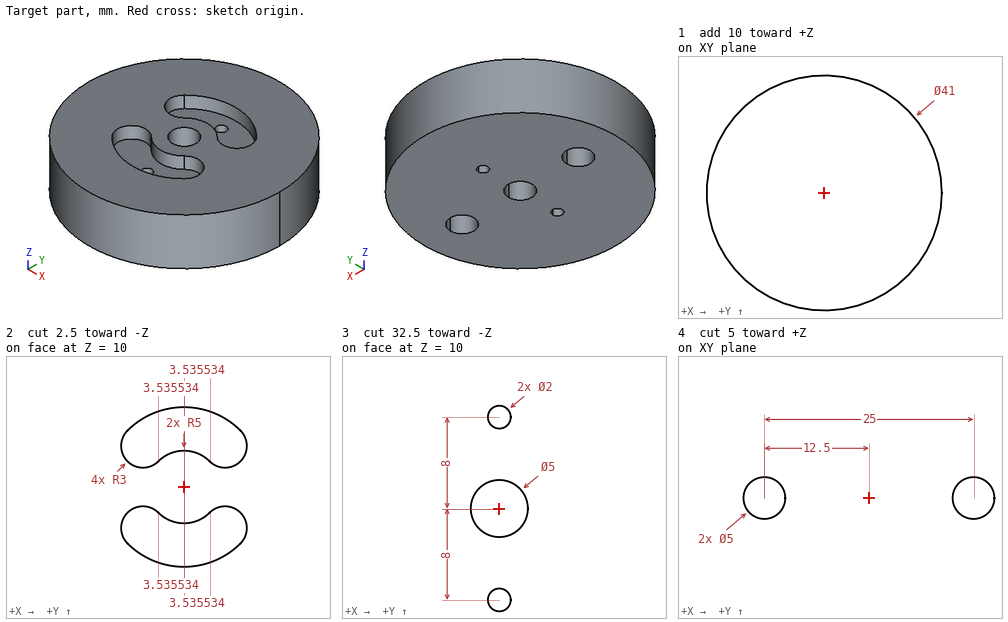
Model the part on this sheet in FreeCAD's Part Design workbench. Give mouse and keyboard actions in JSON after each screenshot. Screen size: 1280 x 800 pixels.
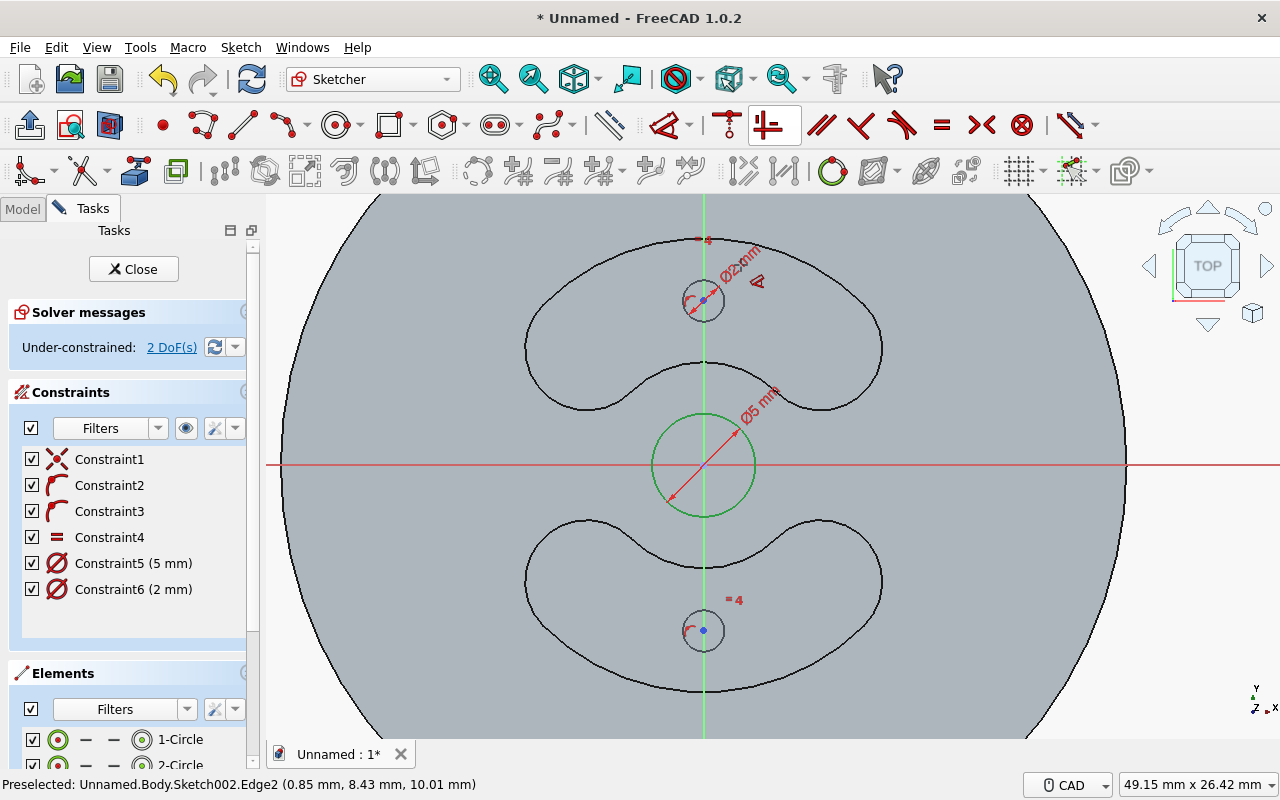
{"action": "left_click", "coordinate": [704, 301]}
{"action": "left_click", "coordinate": [738, 383]}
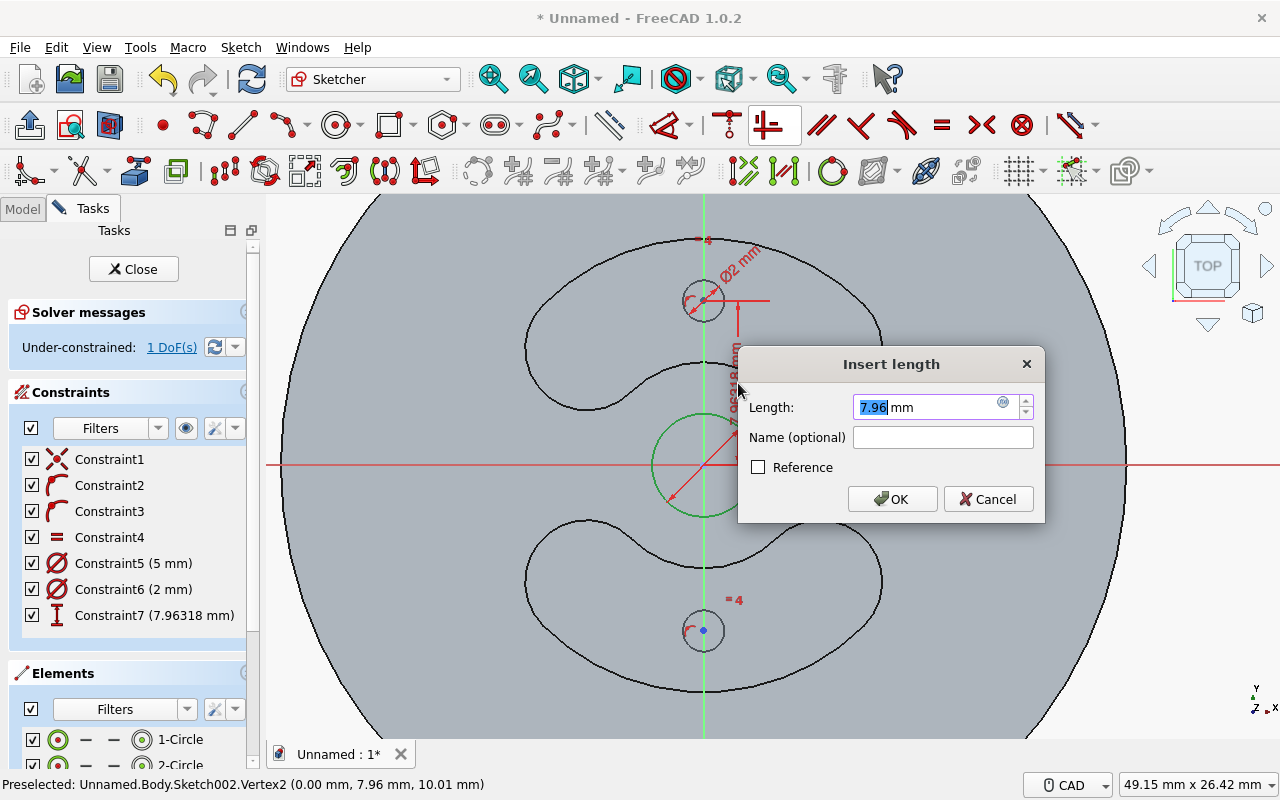
{"action": "type", "text": "8"}
{"action": "key", "text": "Return"}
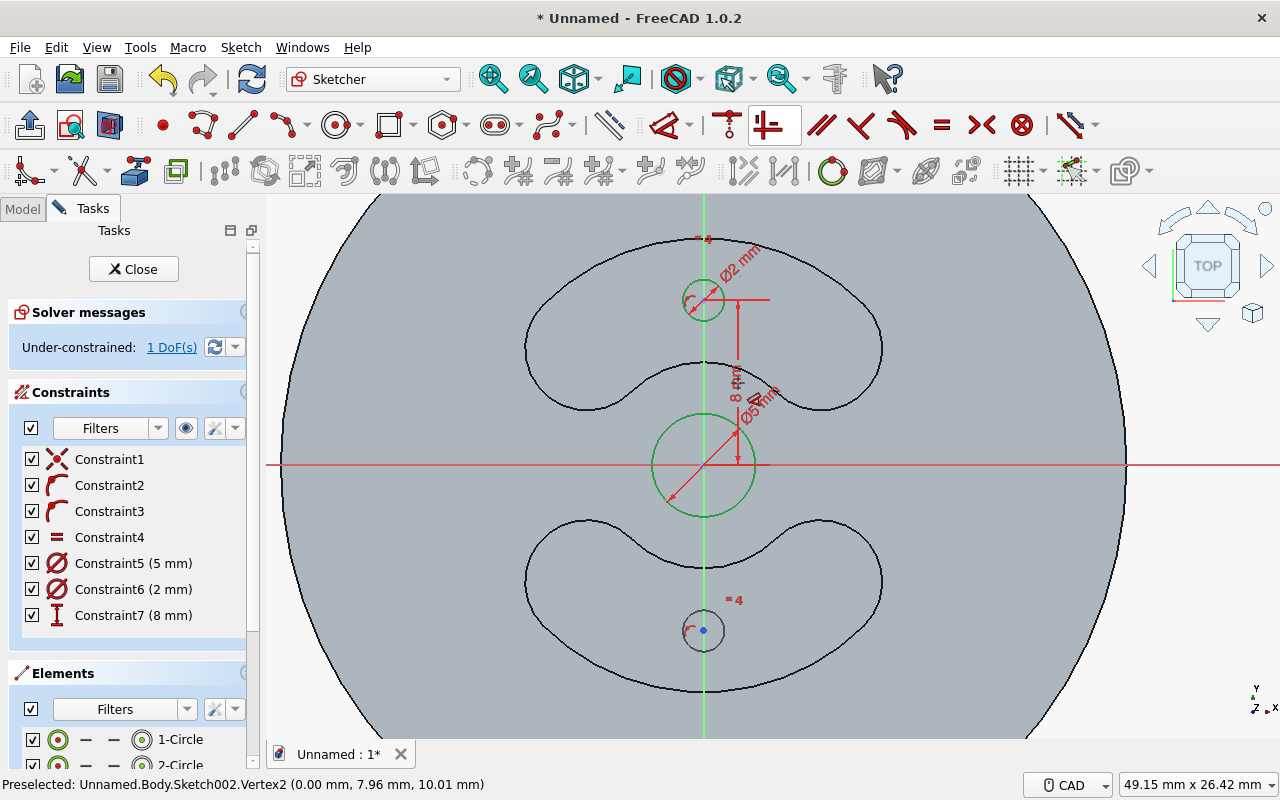
{"action": "left_click", "coordinate": [704, 631]}
{"action": "left_click", "coordinate": [738, 548]}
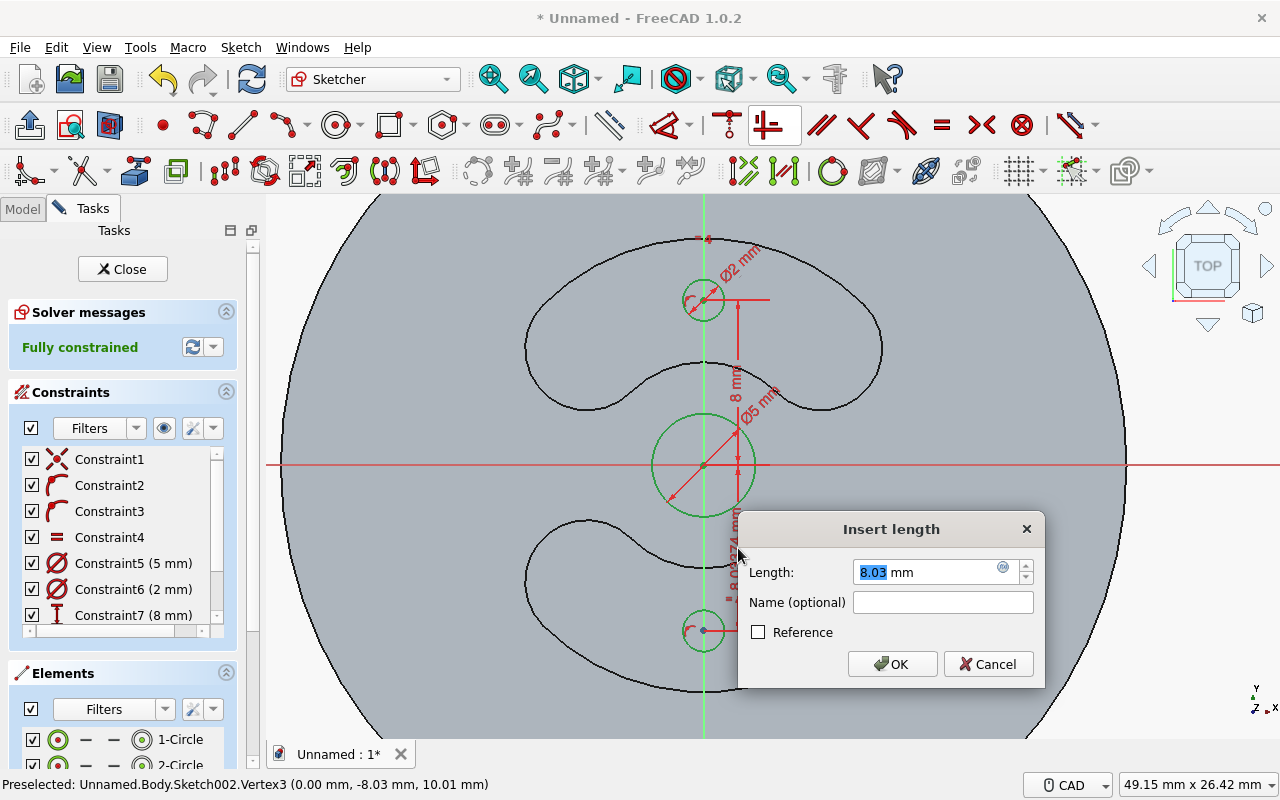
{"action": "type", "text": "8"}
{"action": "key", "text": "Return"}
{"action": "key", "text": "Escape"}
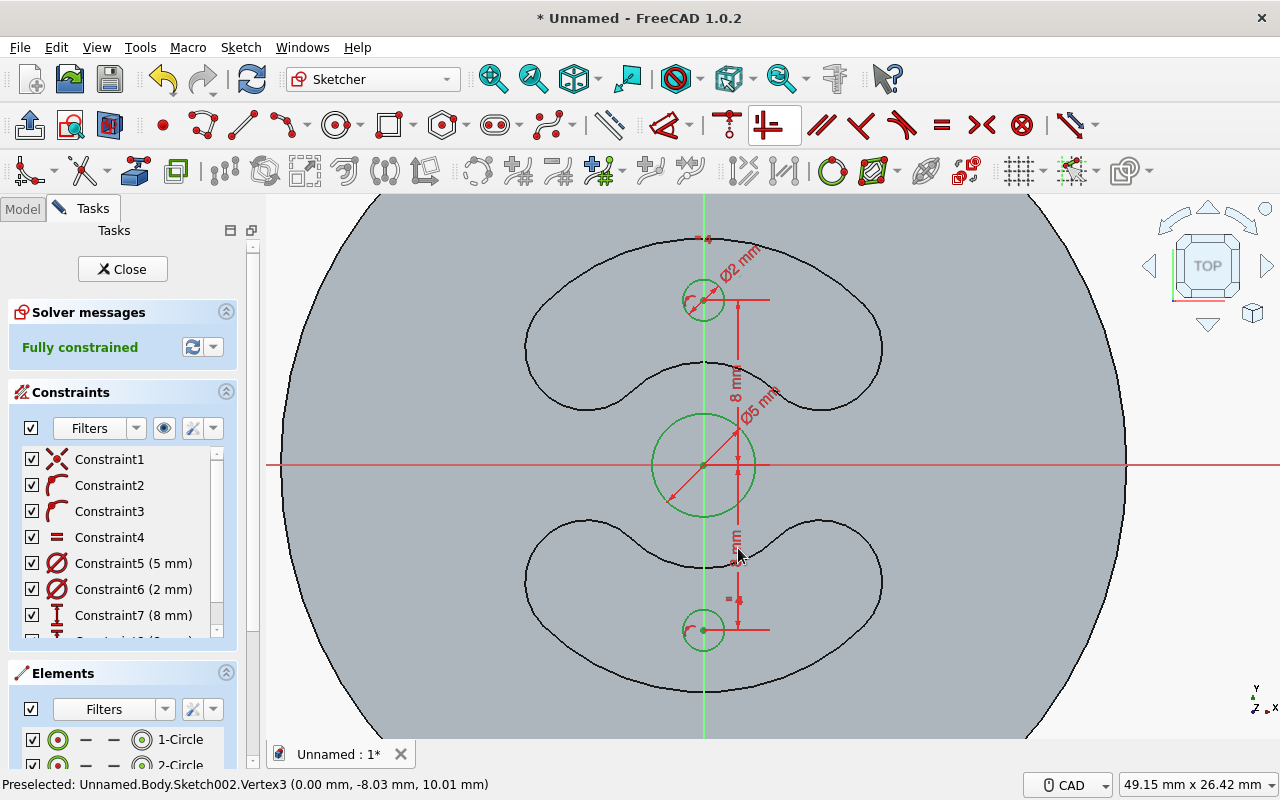
{"action": "left_click", "coordinate": [123, 269]}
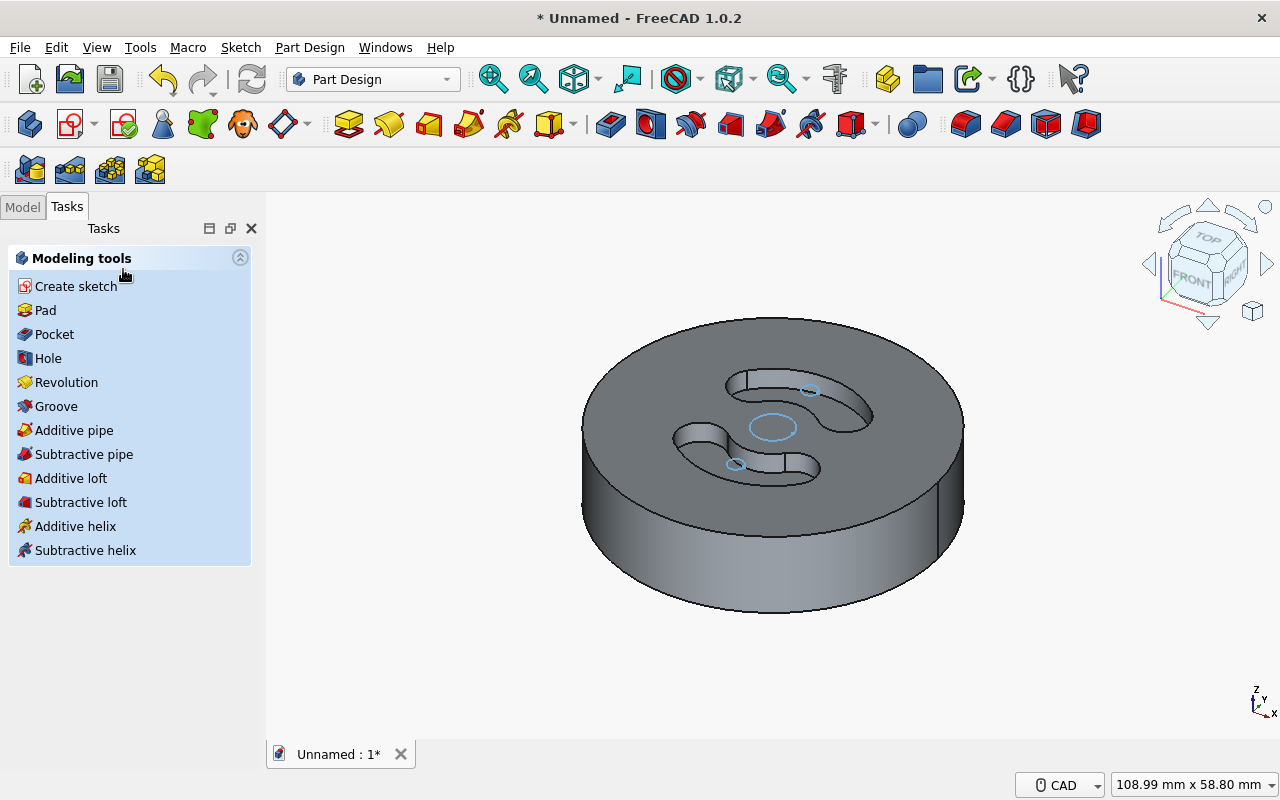
{"action": "left_click", "coordinate": [612, 124]}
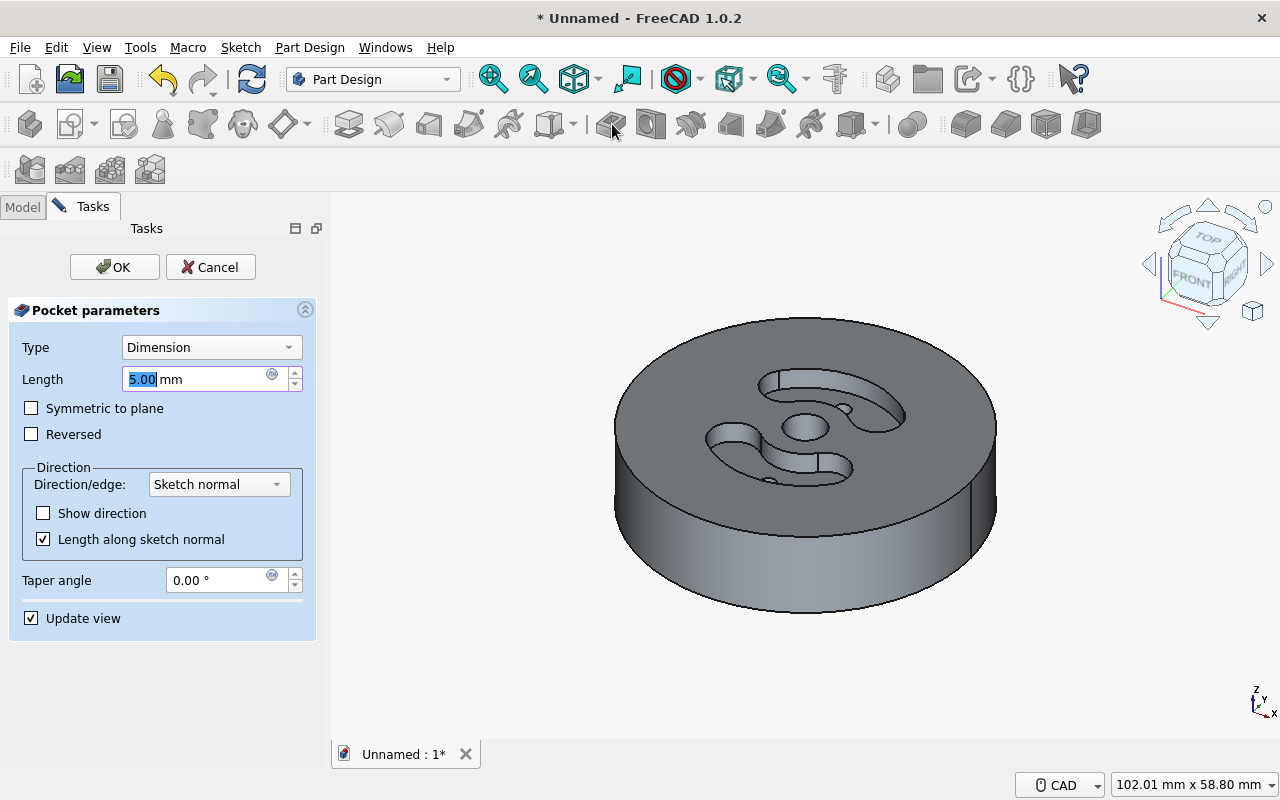
{"action": "type", "text": "32.5"}
{"action": "key", "text": "Tab"}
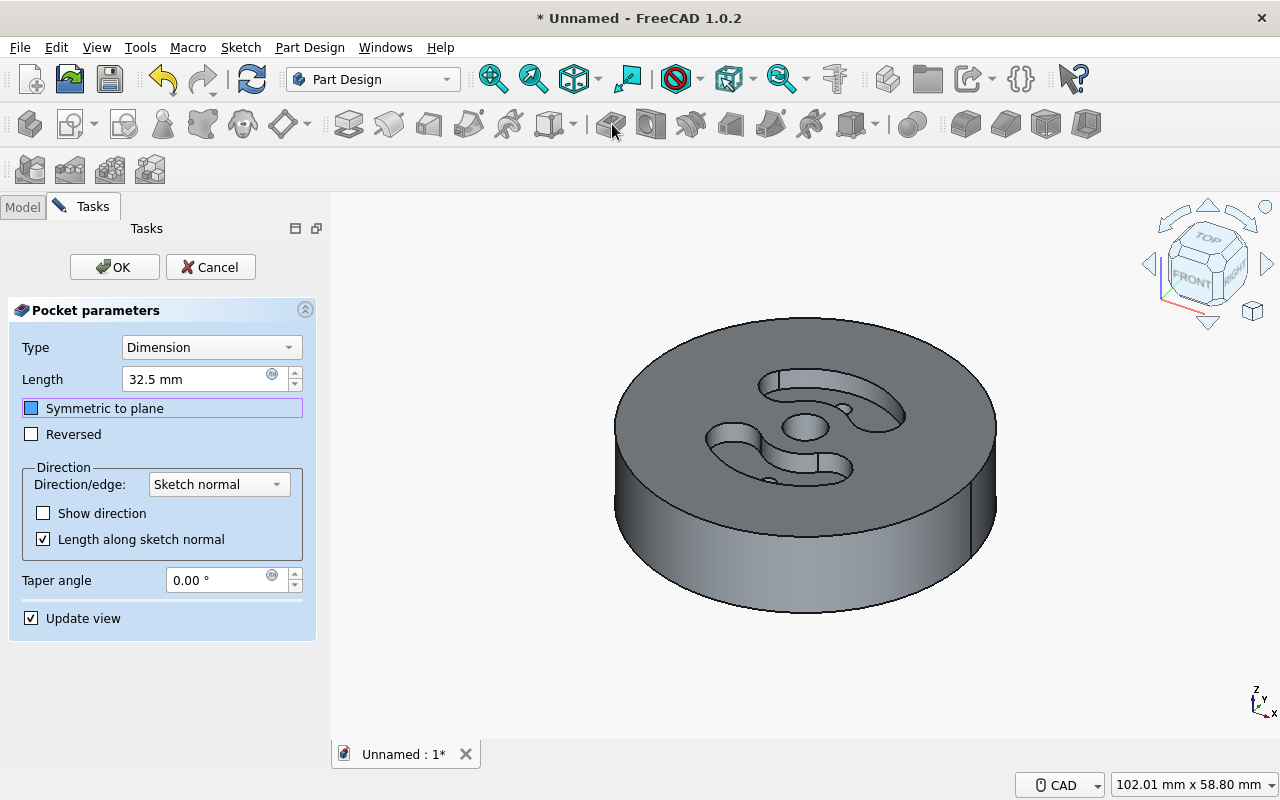
{"action": "left_click", "coordinate": [115, 267]}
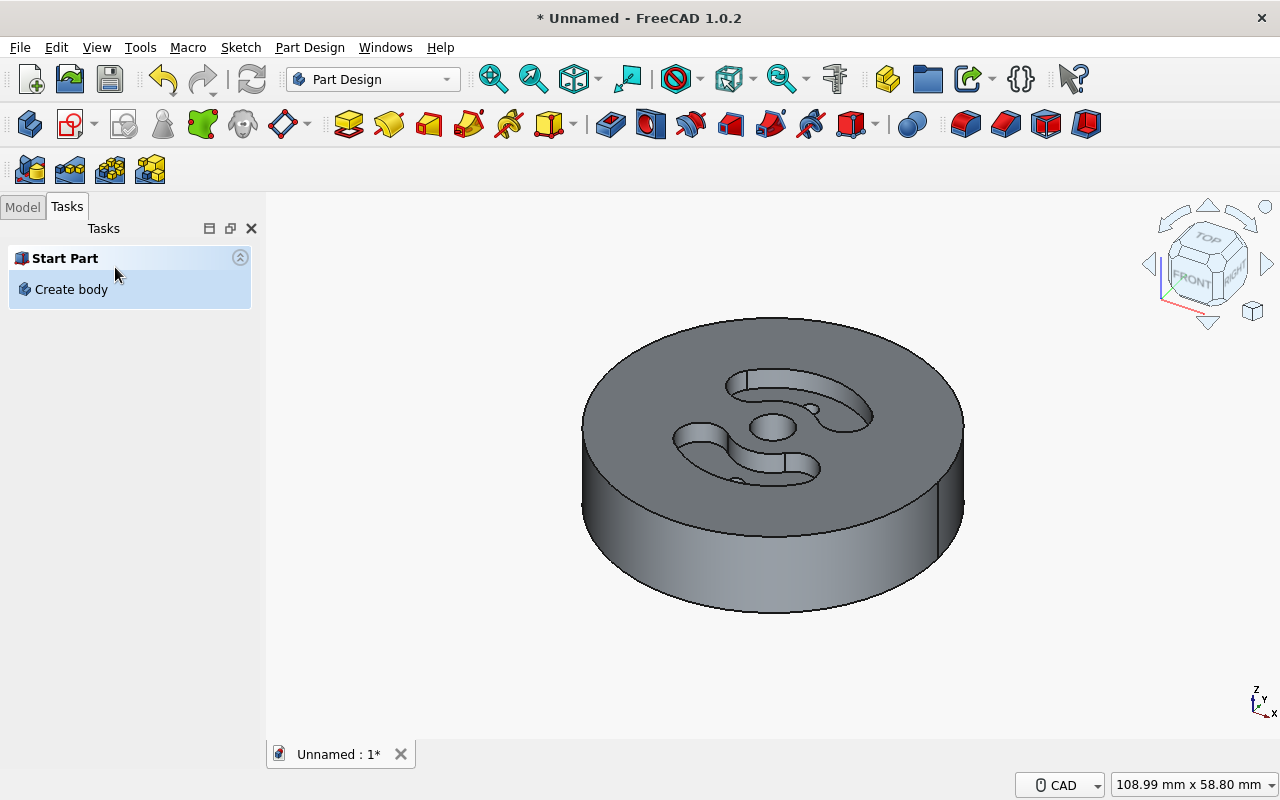
{"action": "left_click", "coordinate": [70, 124]}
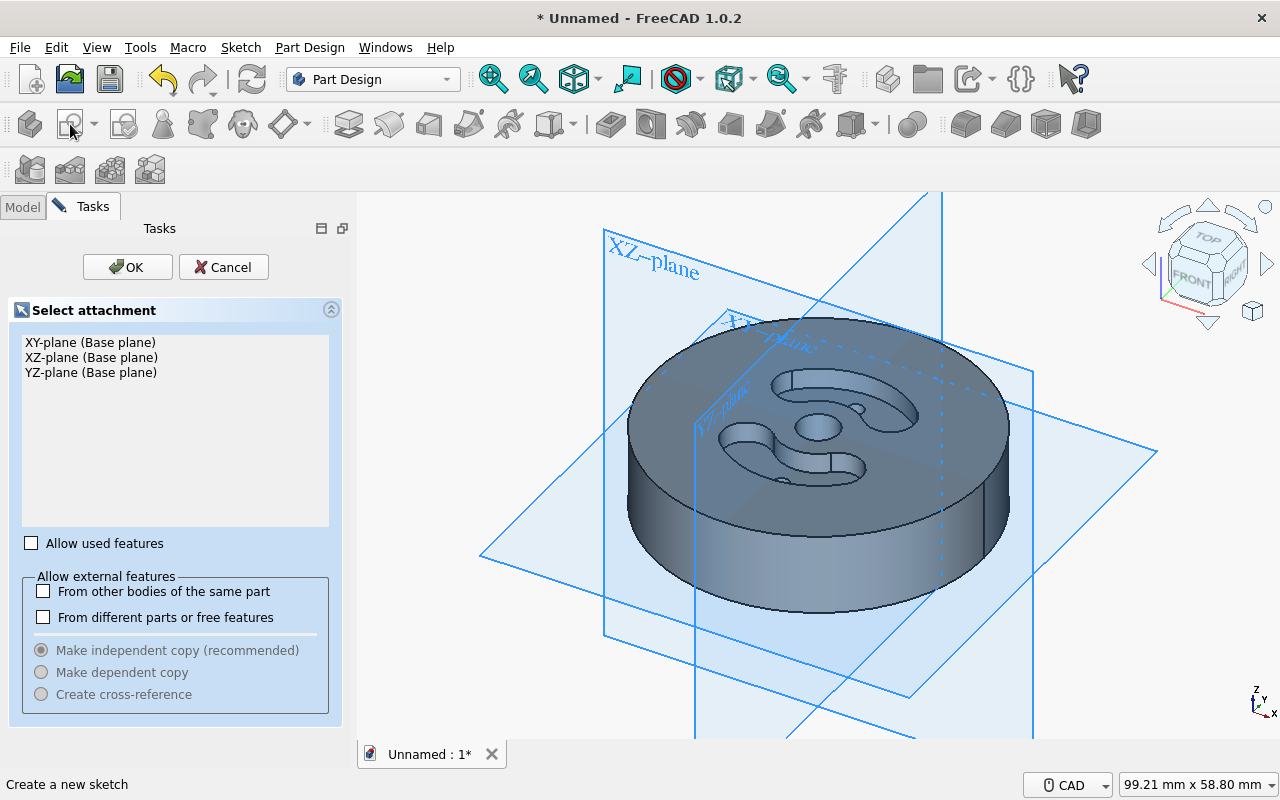
{"action": "left_click", "coordinate": [82, 342]}